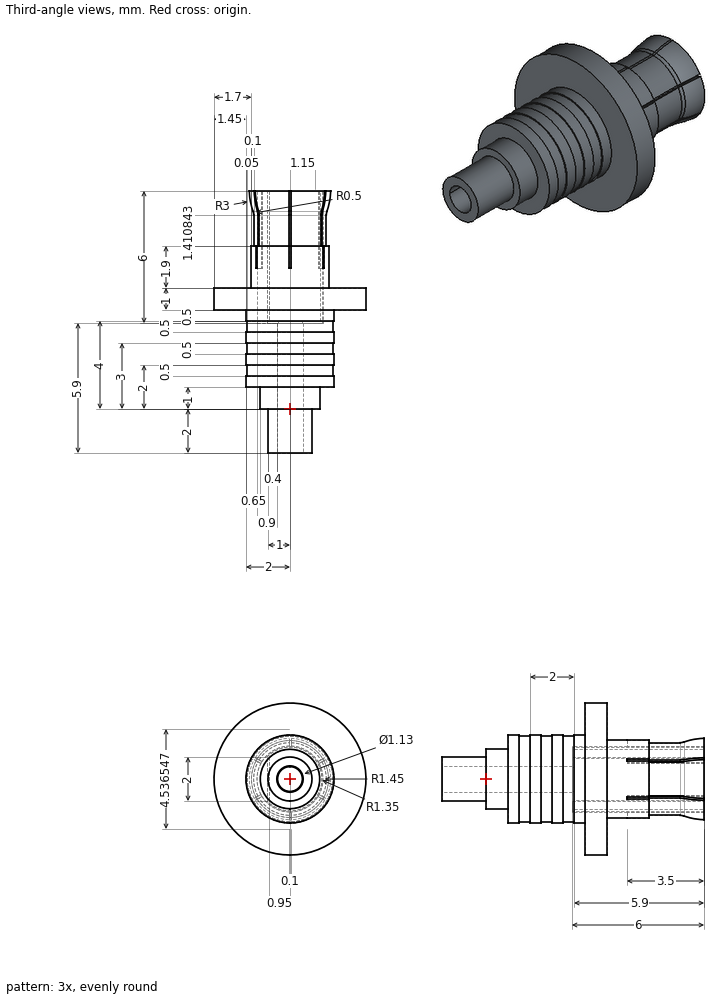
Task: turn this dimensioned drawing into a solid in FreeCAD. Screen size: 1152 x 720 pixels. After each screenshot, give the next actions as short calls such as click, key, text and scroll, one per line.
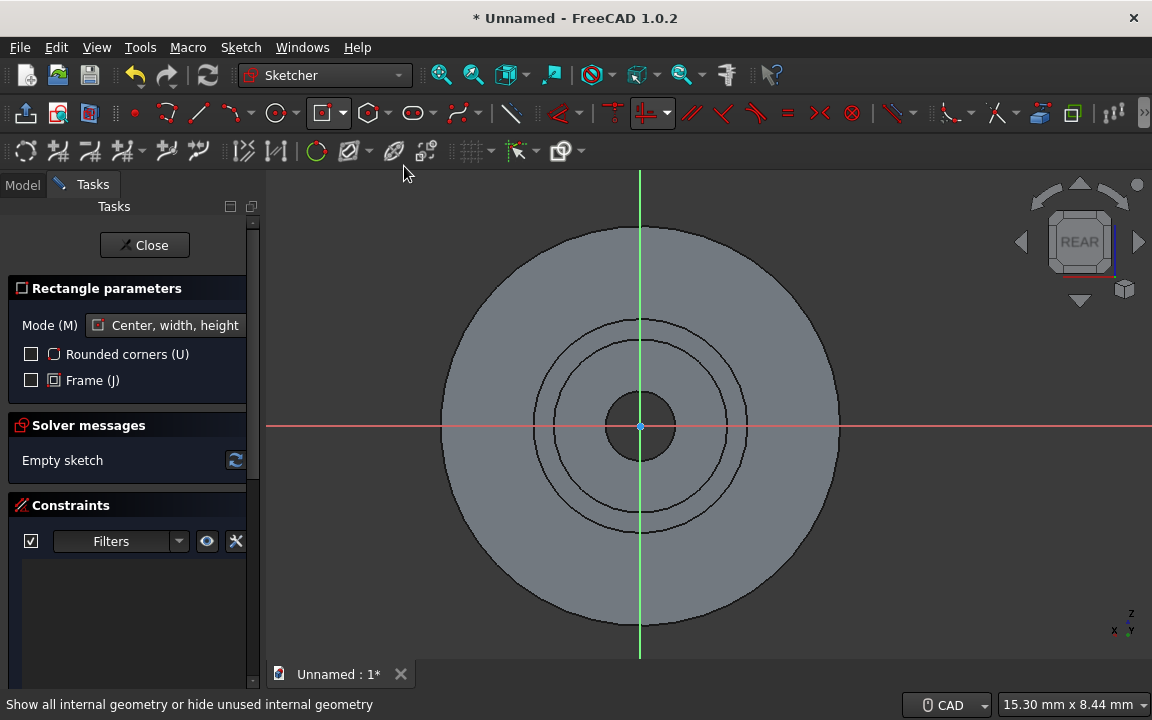
scroll(640, 426, up, 9)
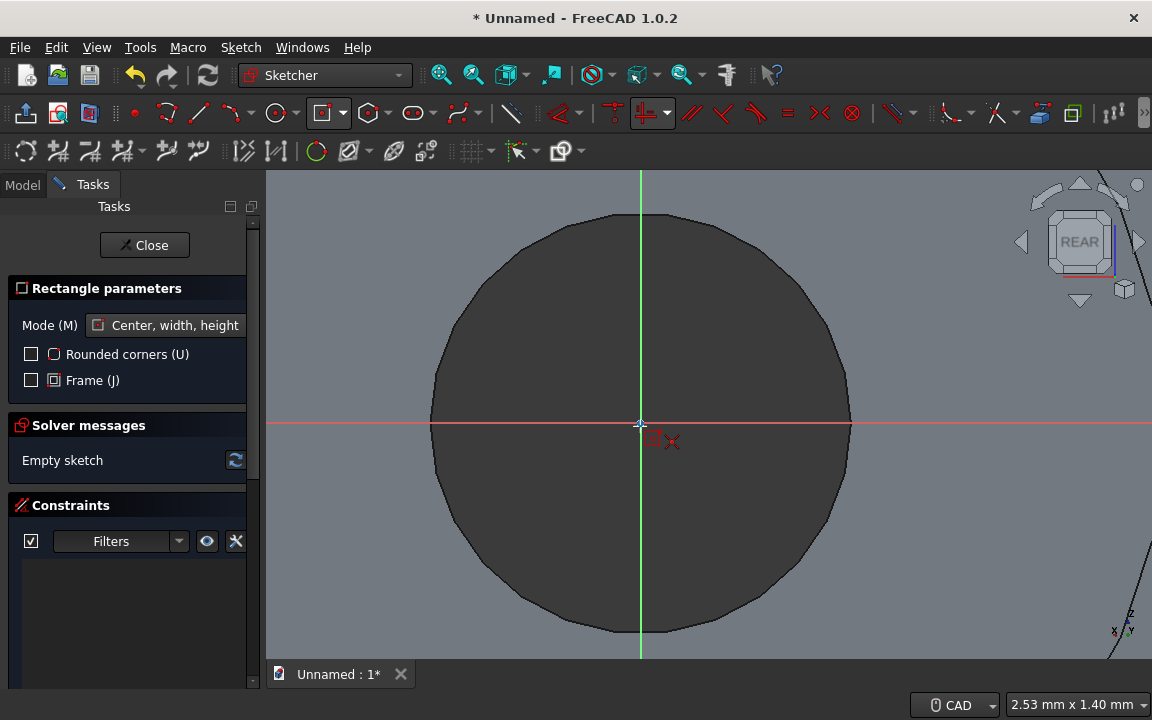
scroll(640, 412, down, 8)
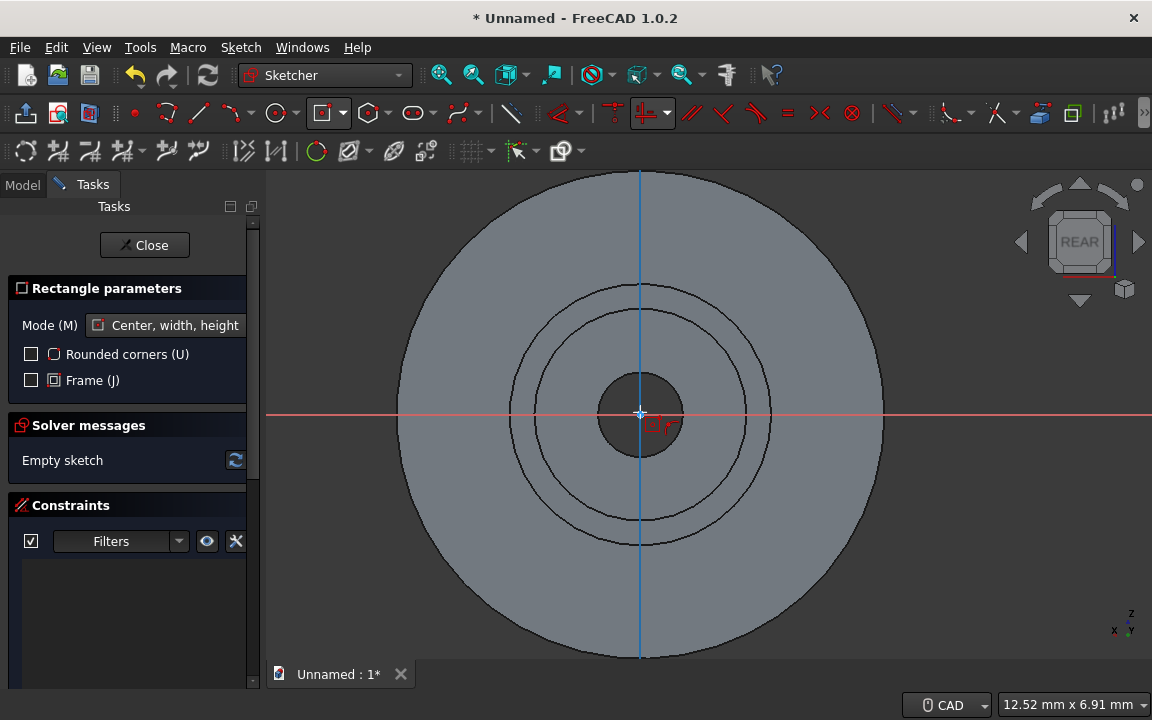
click(640, 415)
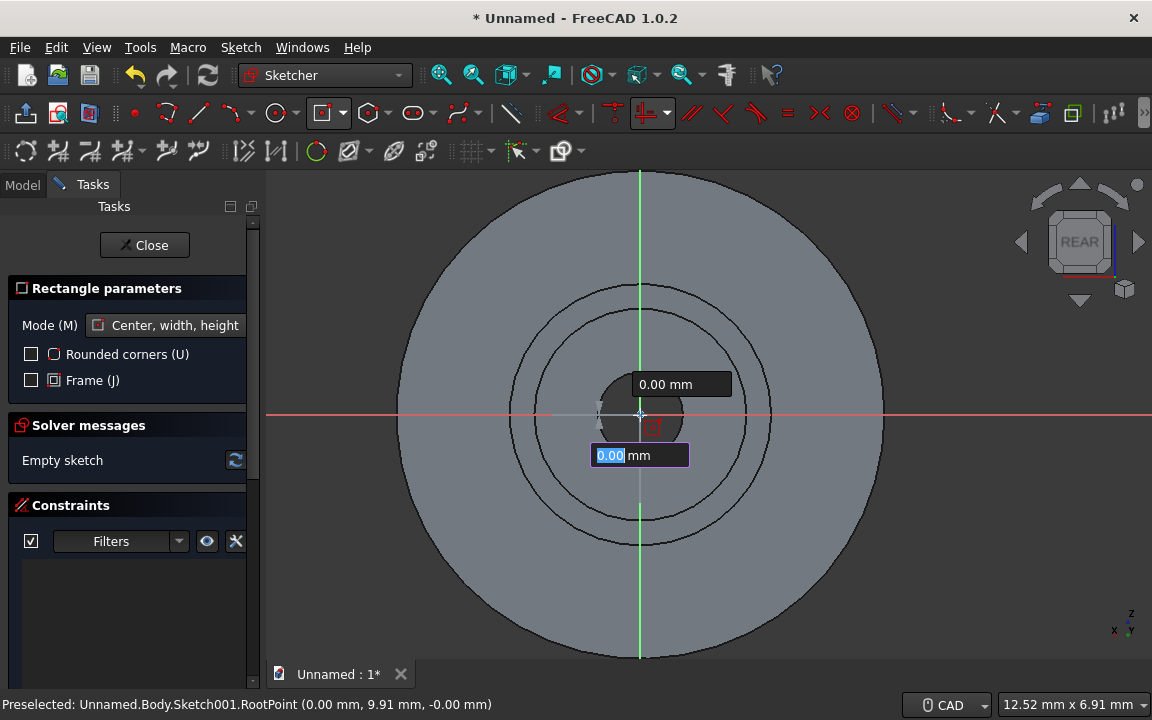
scroll(644, 254, up, 8)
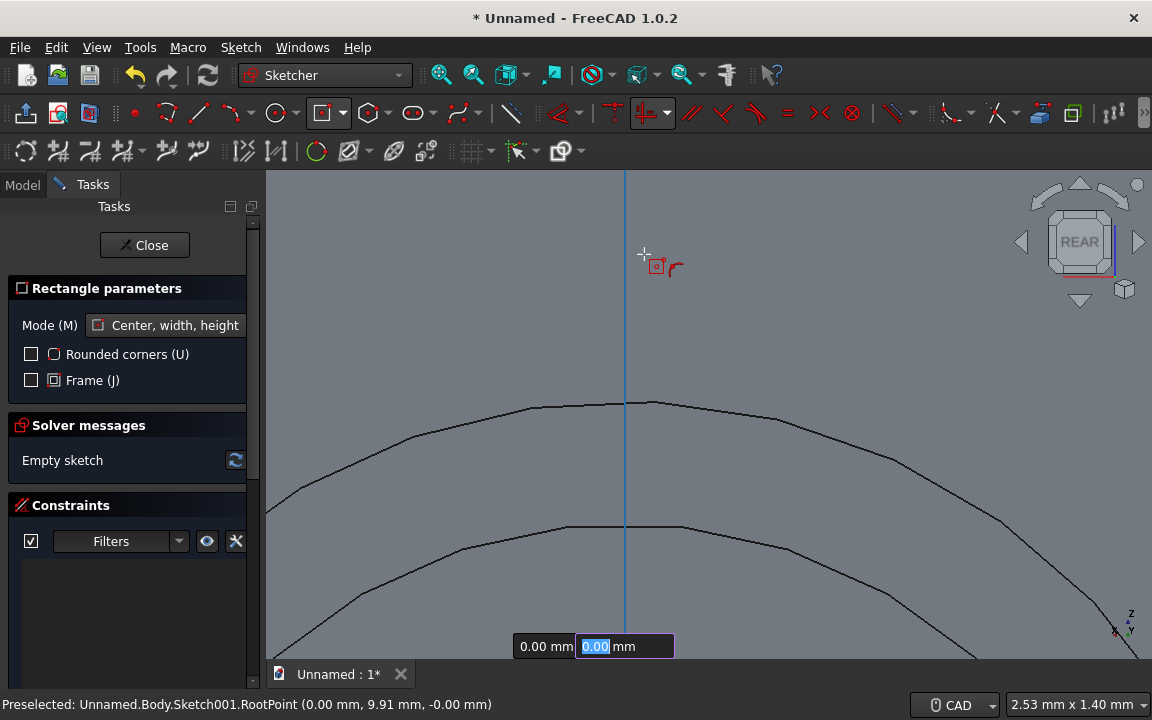
click(642, 254)
key(Escape)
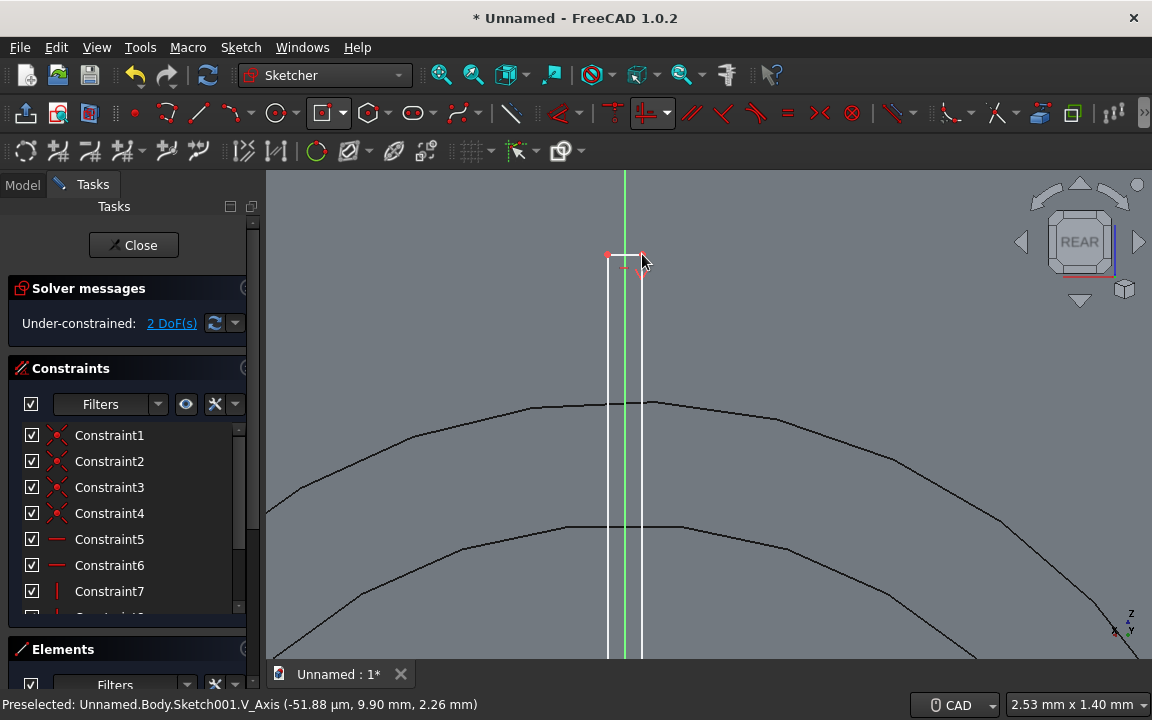
click(558, 114)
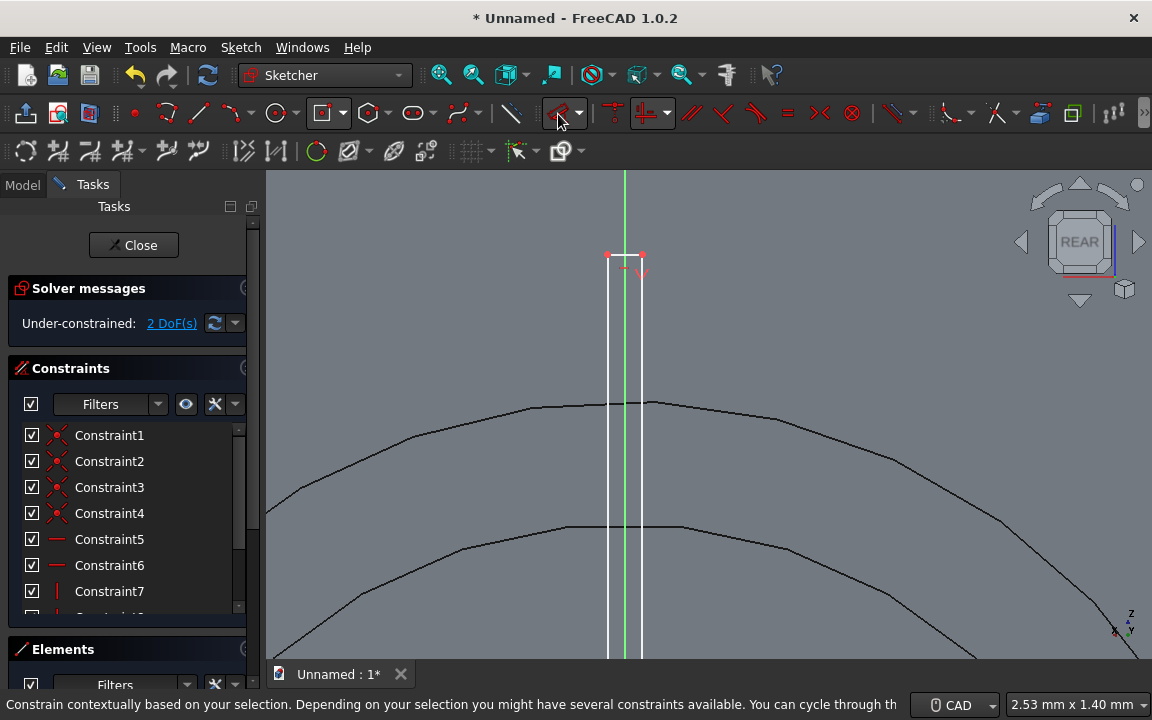
scroll(644, 254, down, 8)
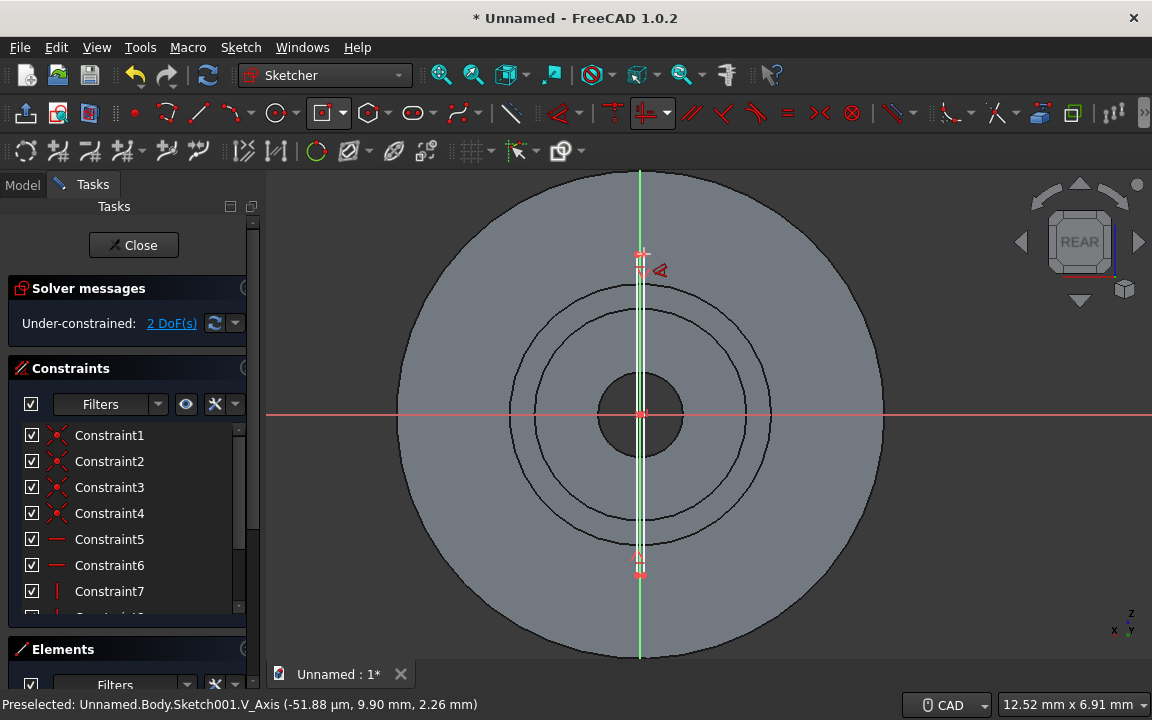
scroll(640, 575, up, 9)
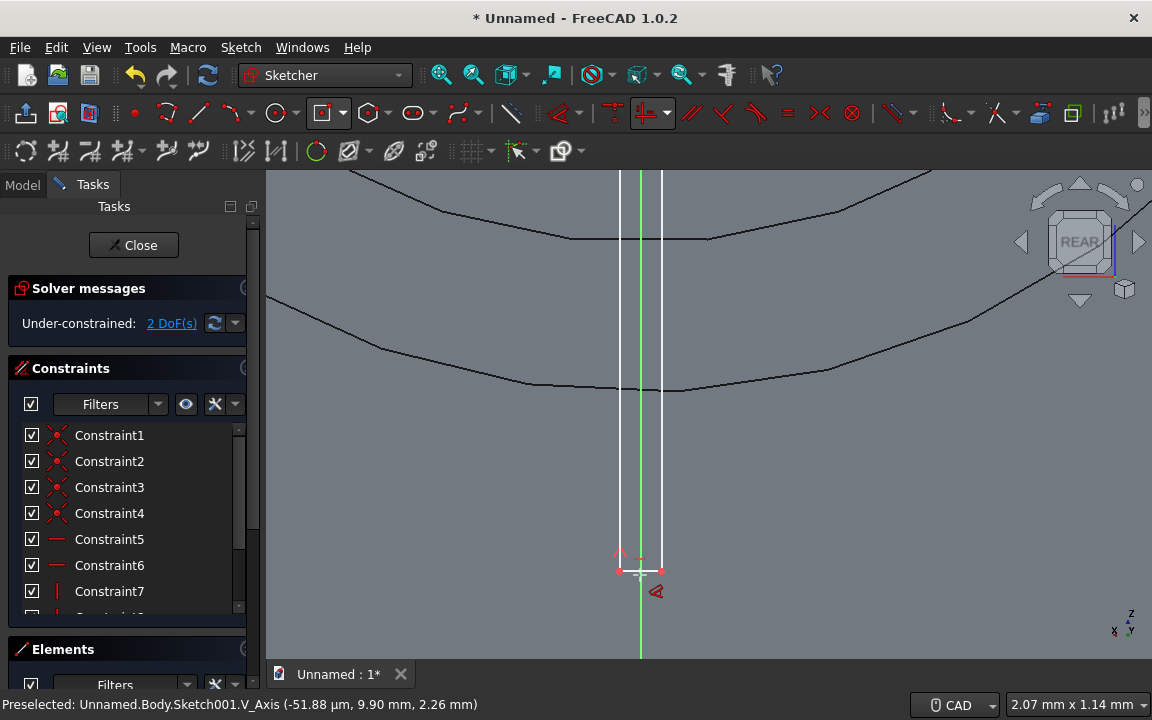
click(637, 571)
click(626, 605)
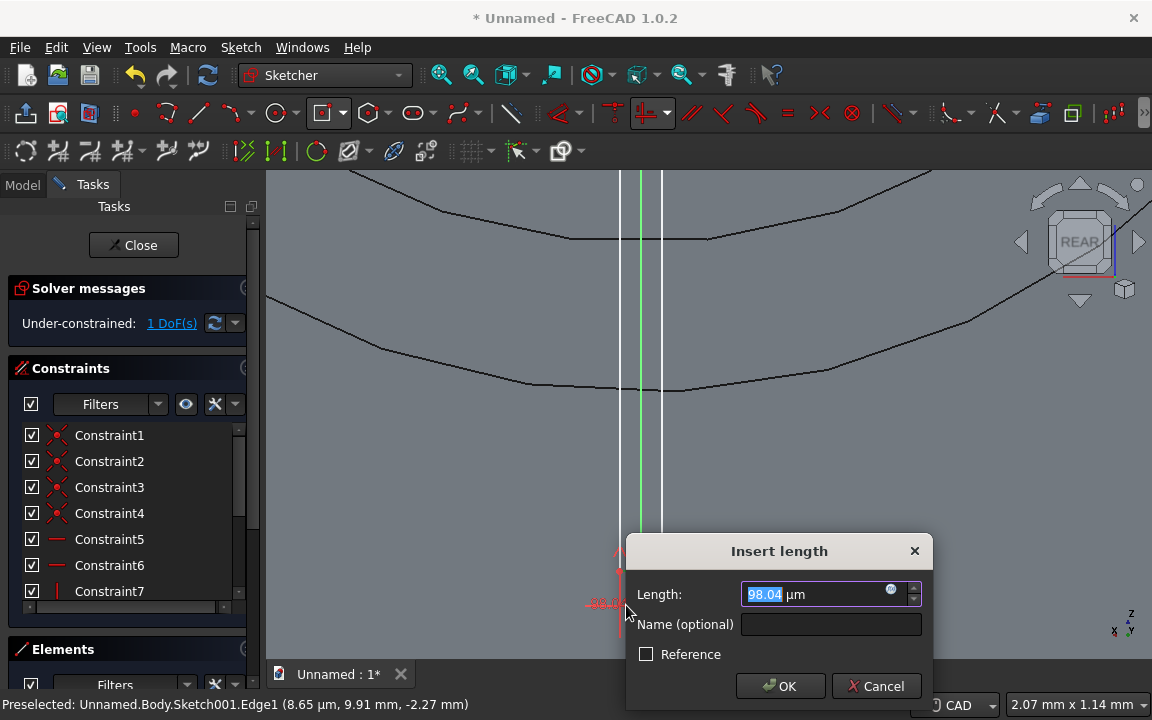
key(ctrl+a)
text(0.1 mm)
key(Return)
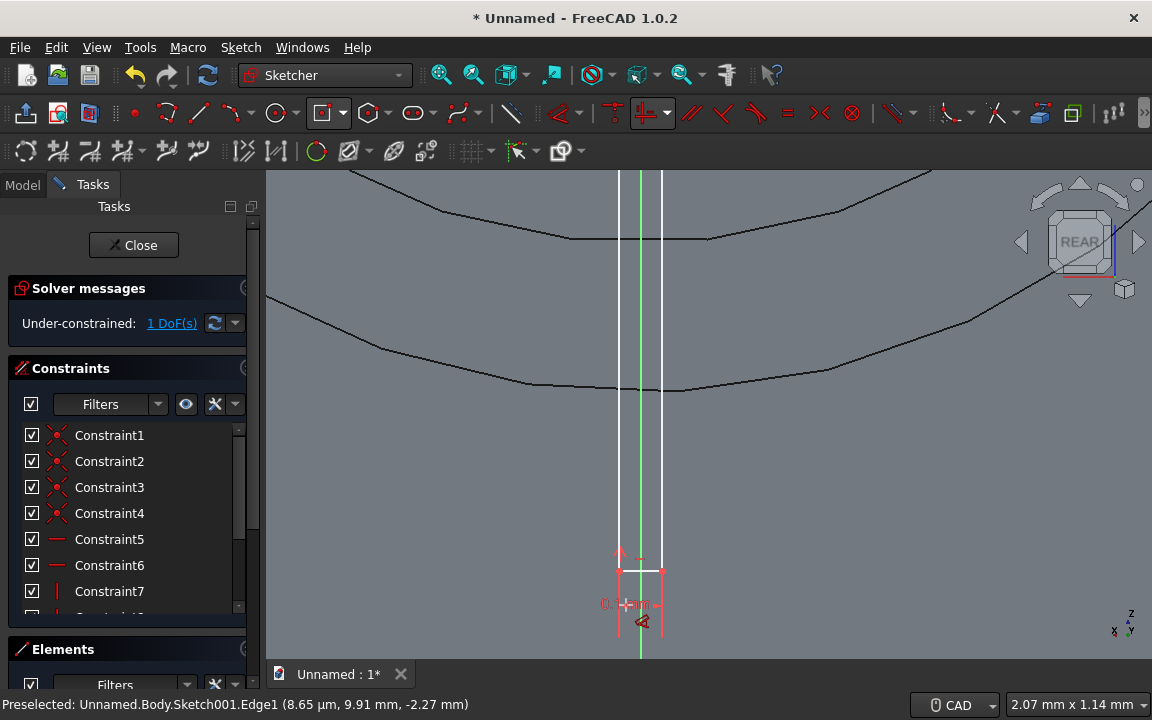
scroll(640, 576, down, 9)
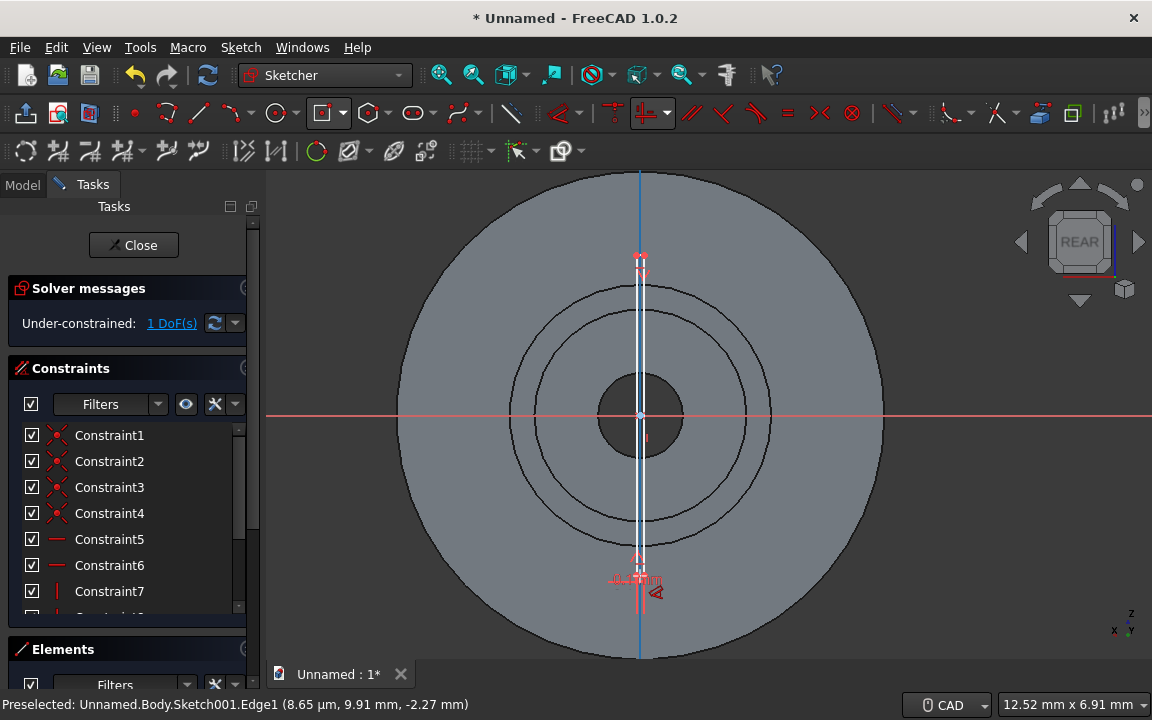
scroll(644, 480, up, 7)